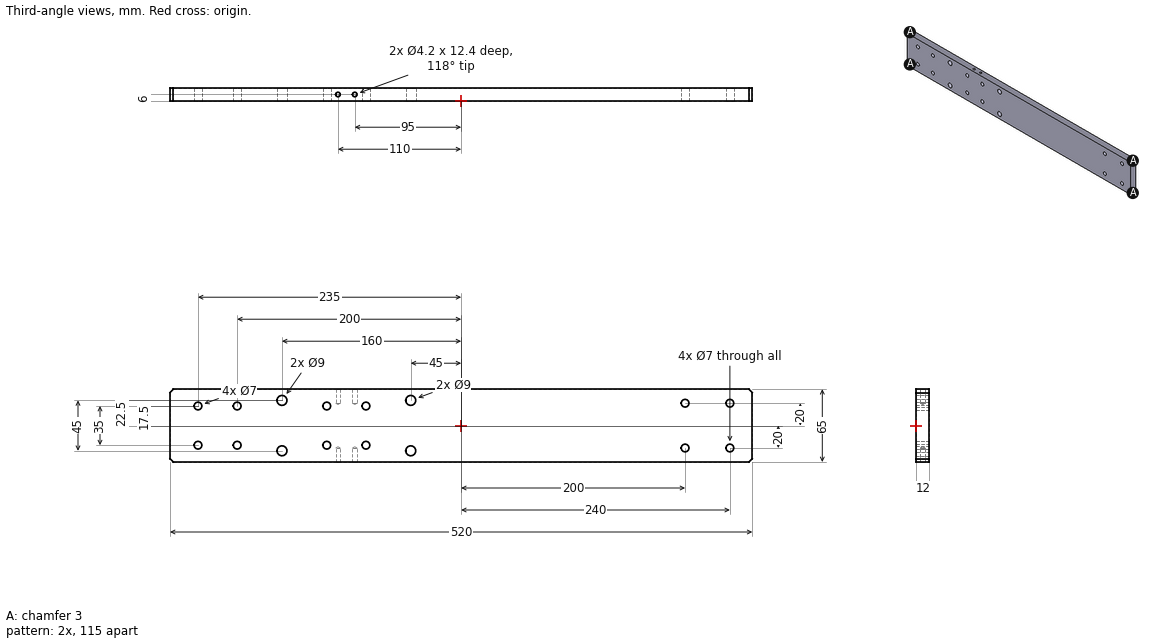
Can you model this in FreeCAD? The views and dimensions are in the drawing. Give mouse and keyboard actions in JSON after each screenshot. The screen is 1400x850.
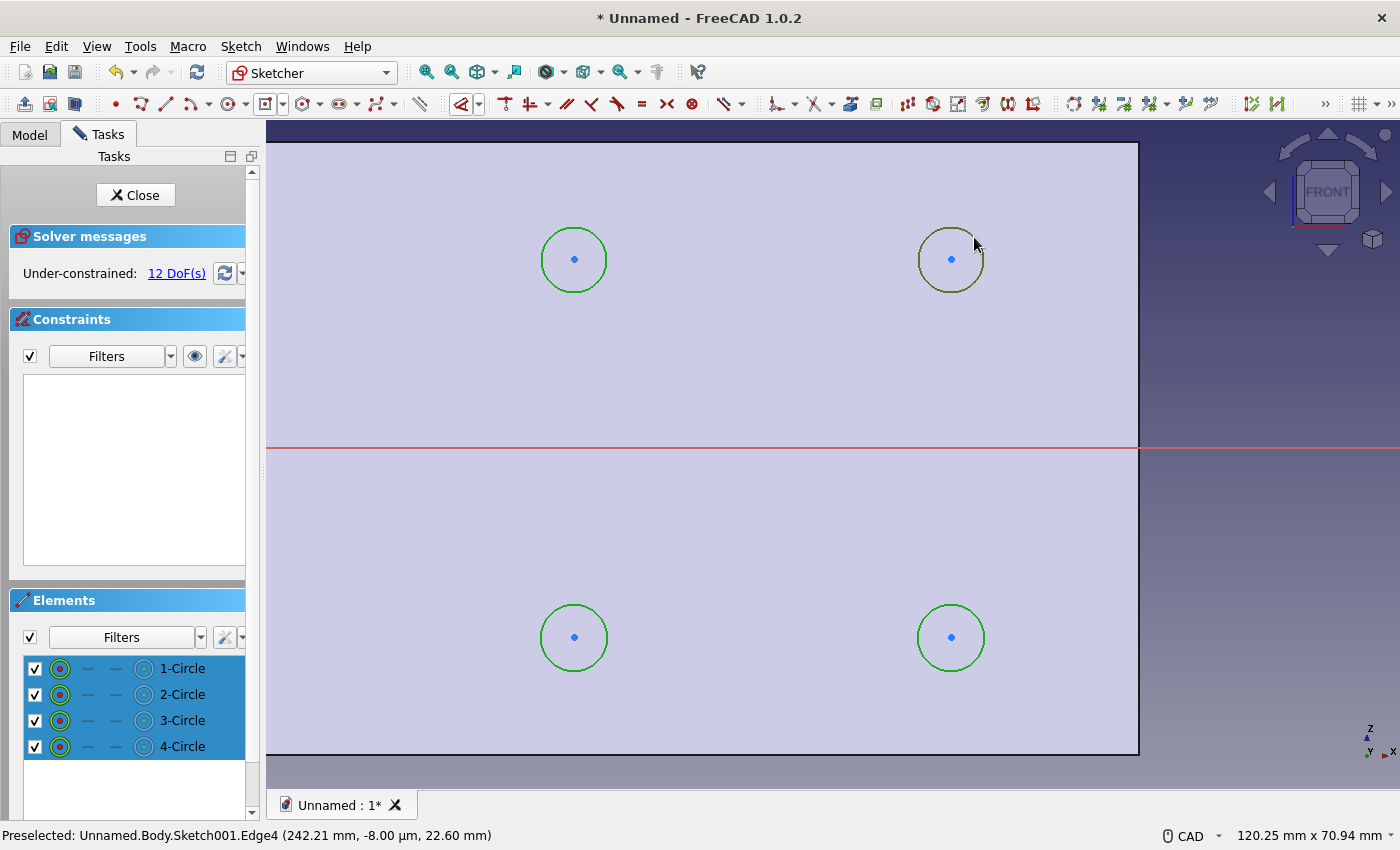
{"action": "left_click", "coordinate": [642, 104]}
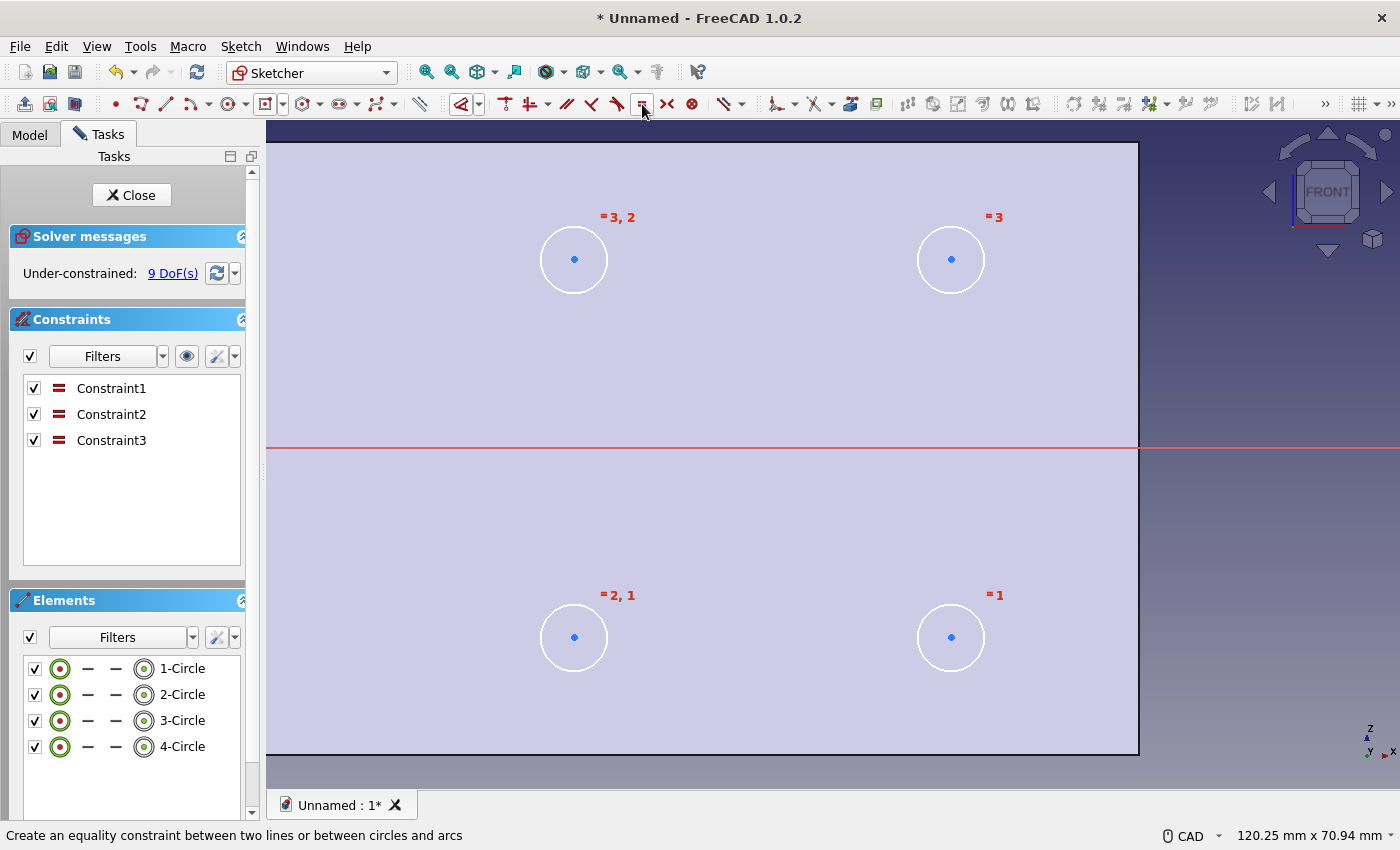
{"action": "left_click", "coordinate": [951, 638]}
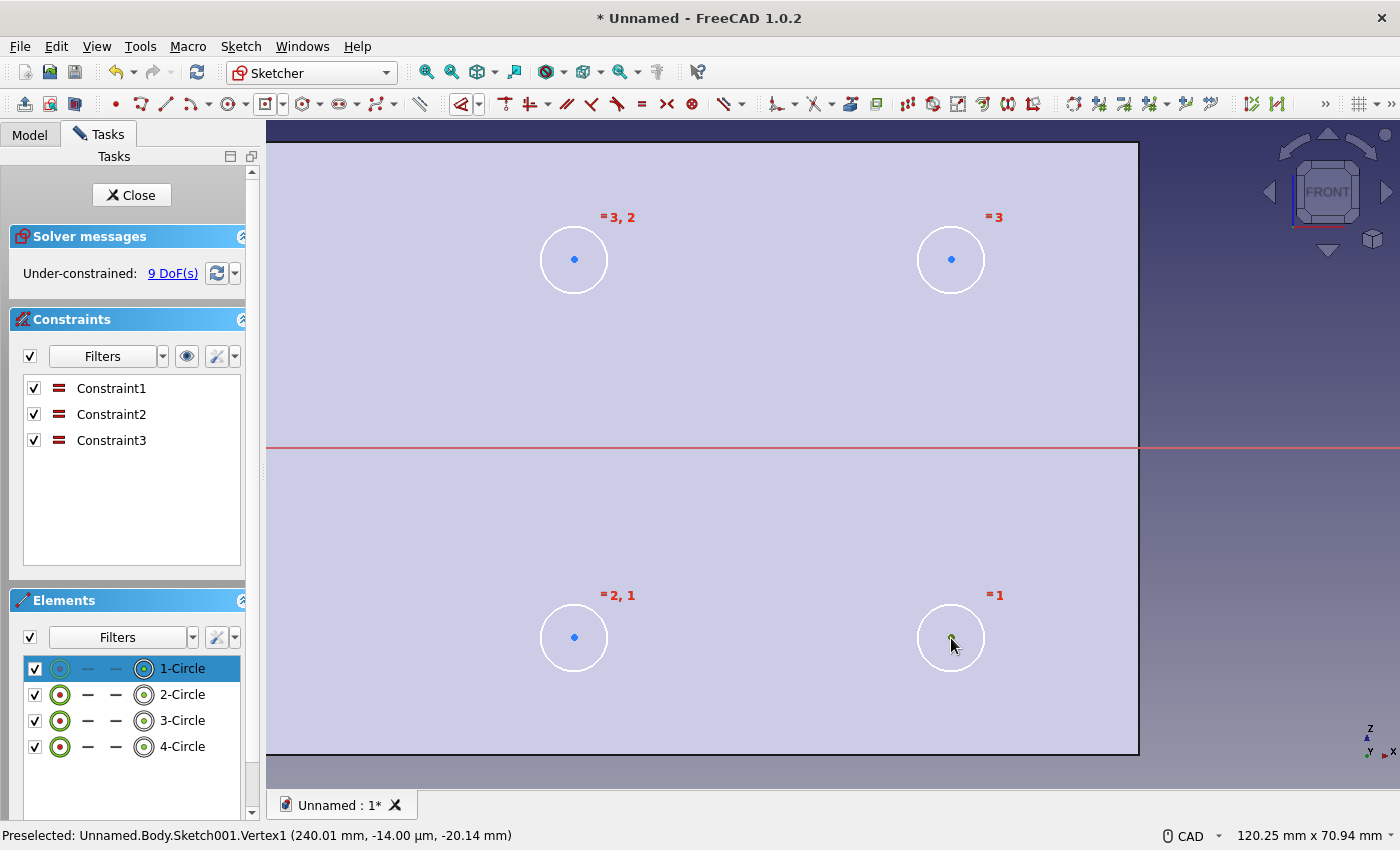
{"action": "left_click", "coordinate": [574, 638]}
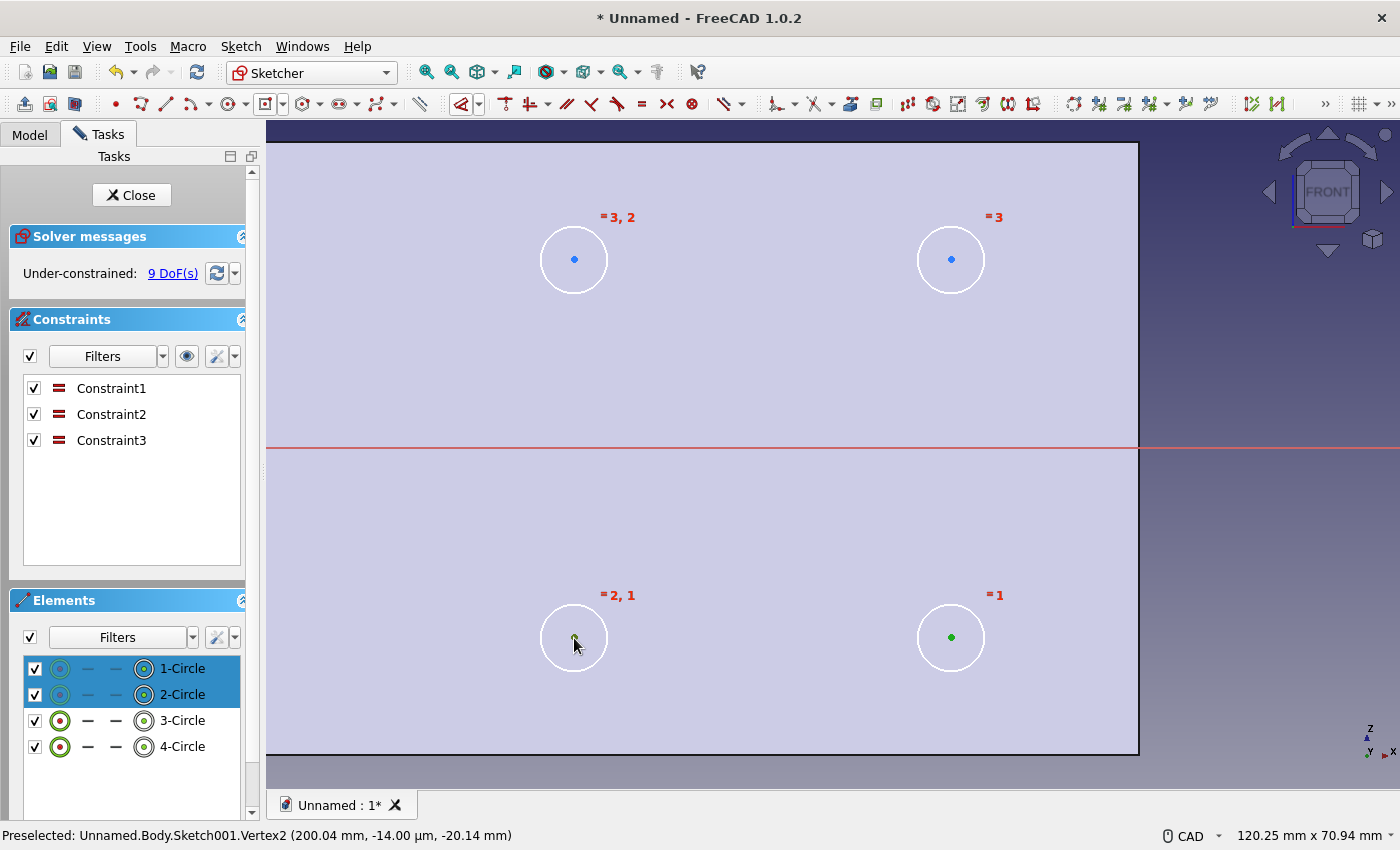
{"action": "key", "text": "h"}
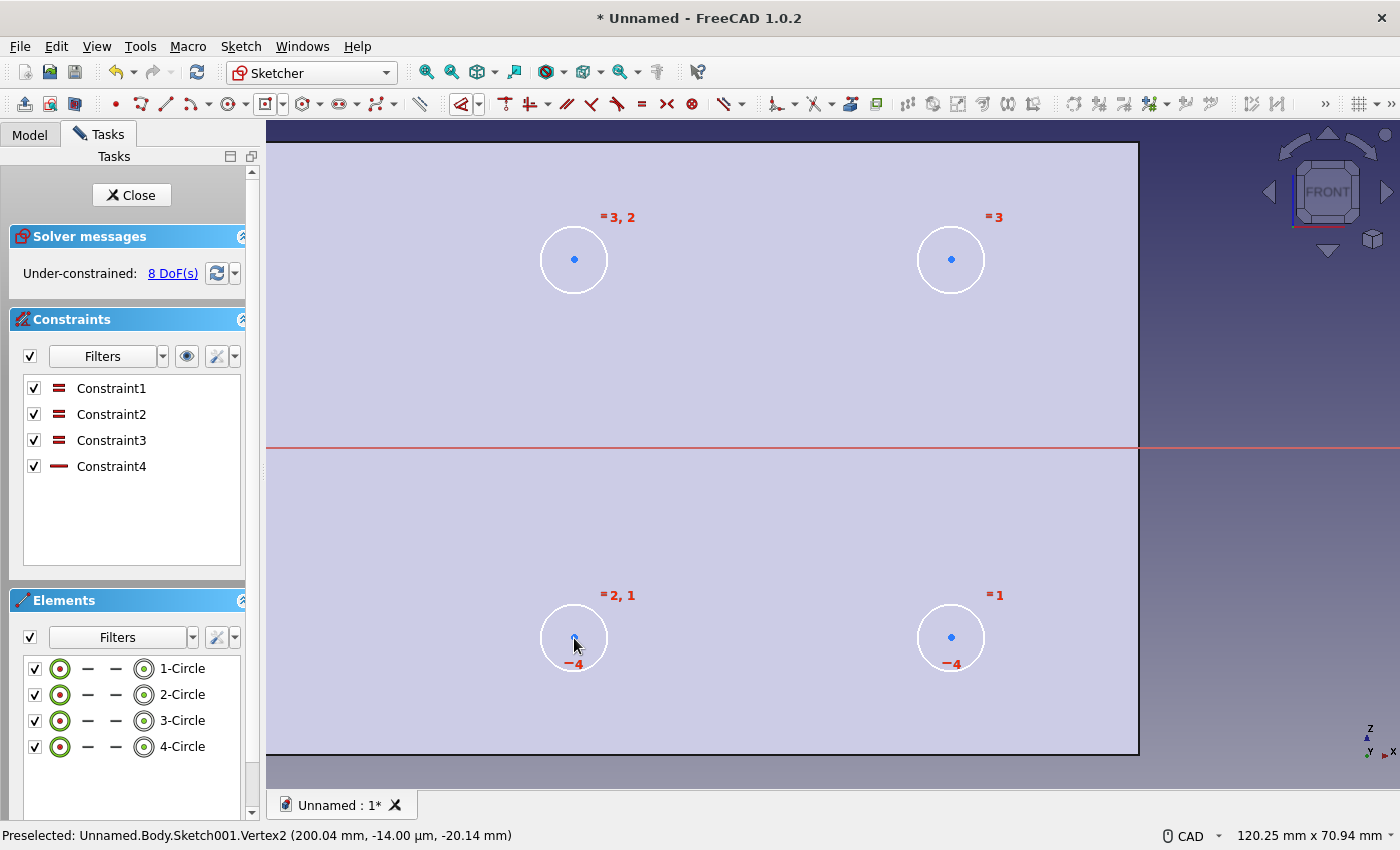
{"action": "left_click", "coordinate": [574, 638]}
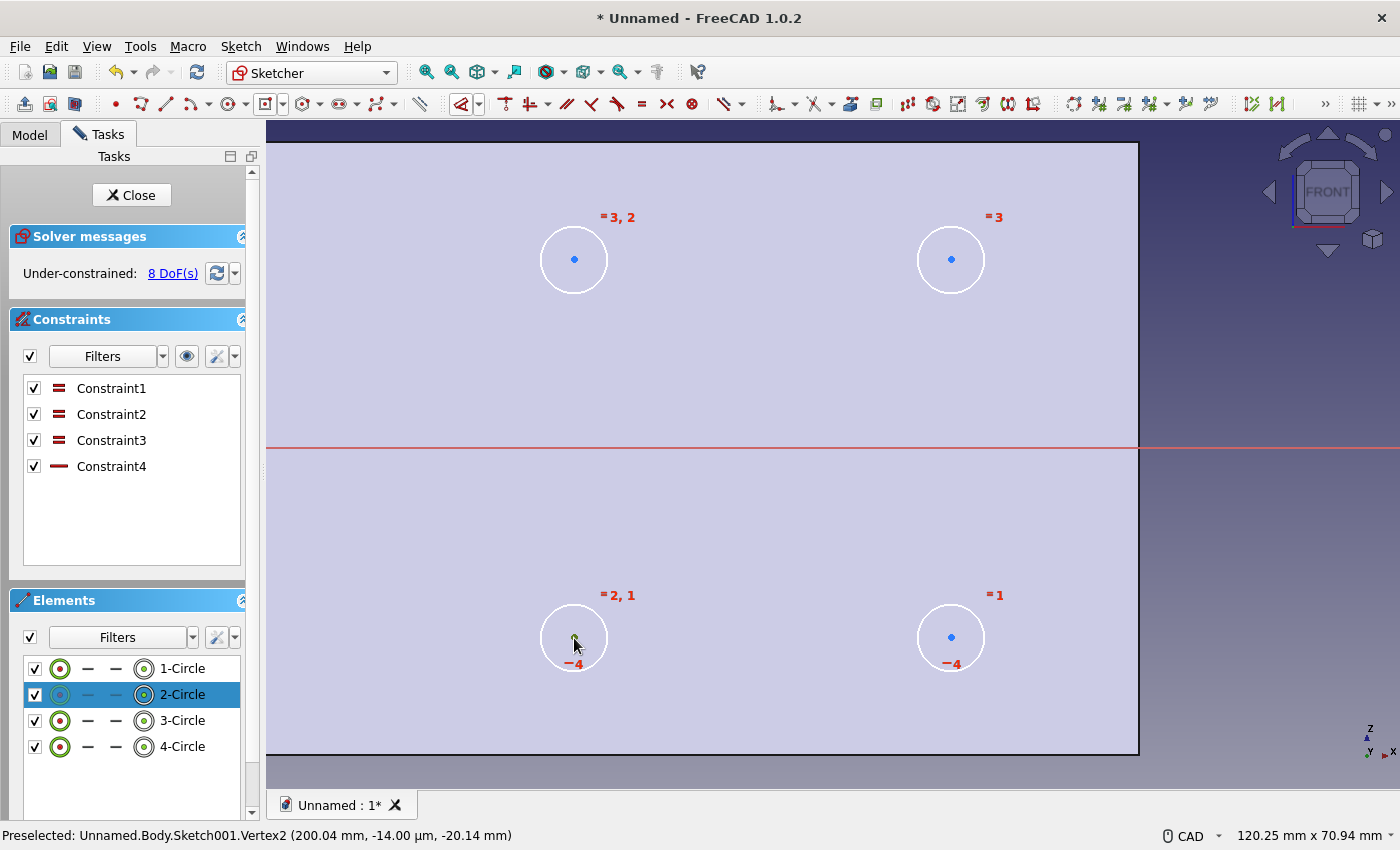
{"action": "left_click", "coordinate": [574, 260]}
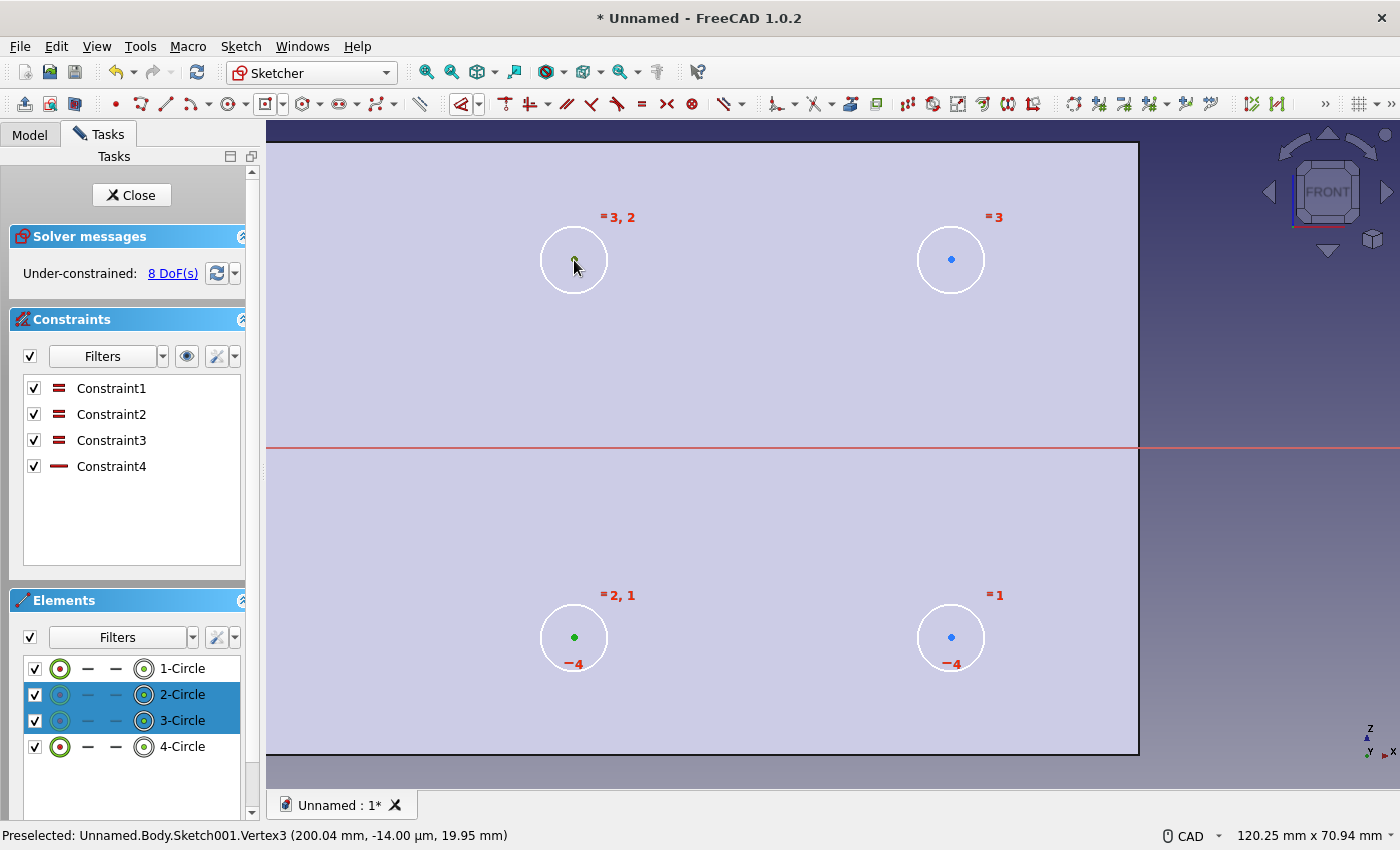
{"action": "key", "text": "v"}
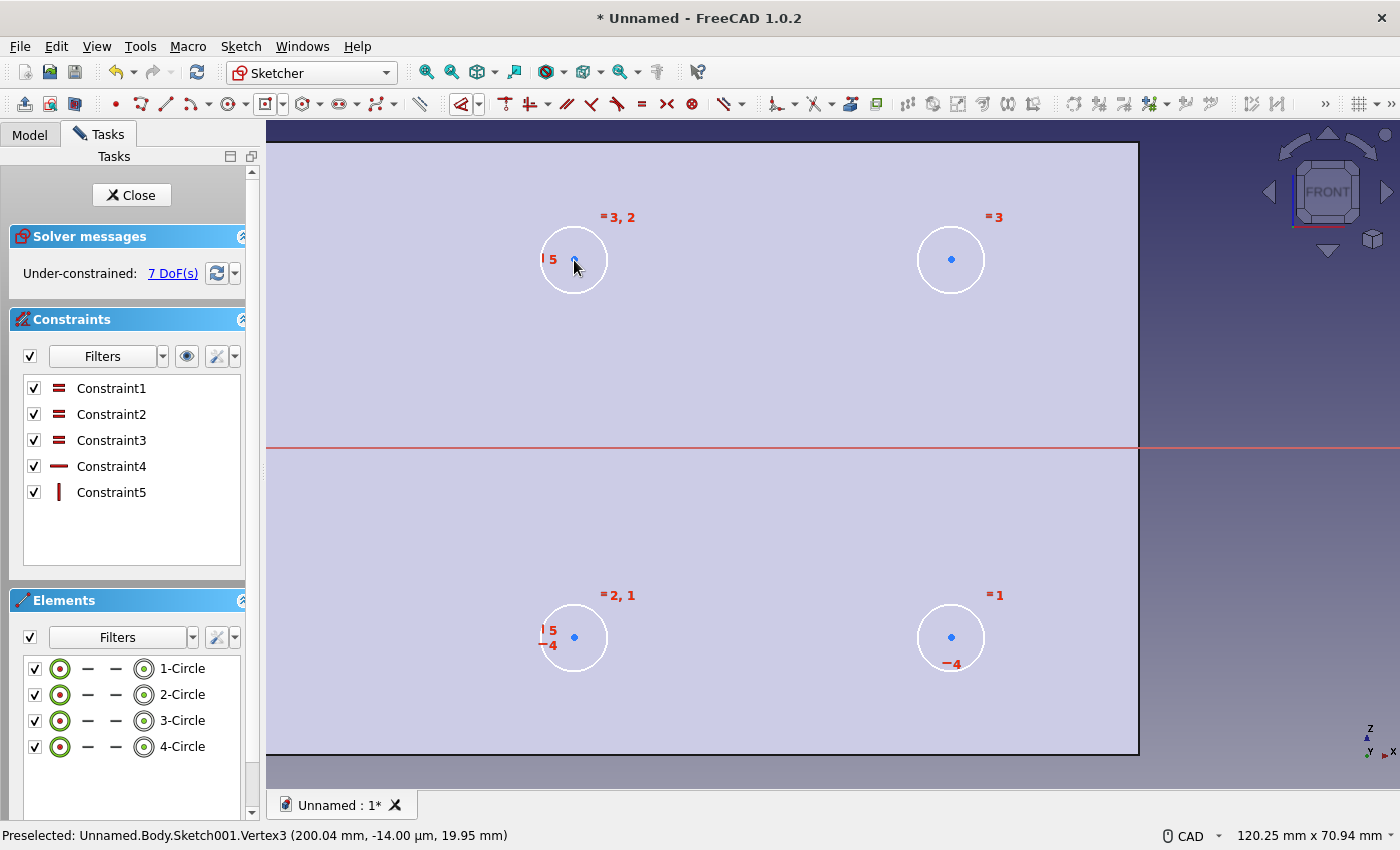
{"action": "left_click", "coordinate": [951, 638]}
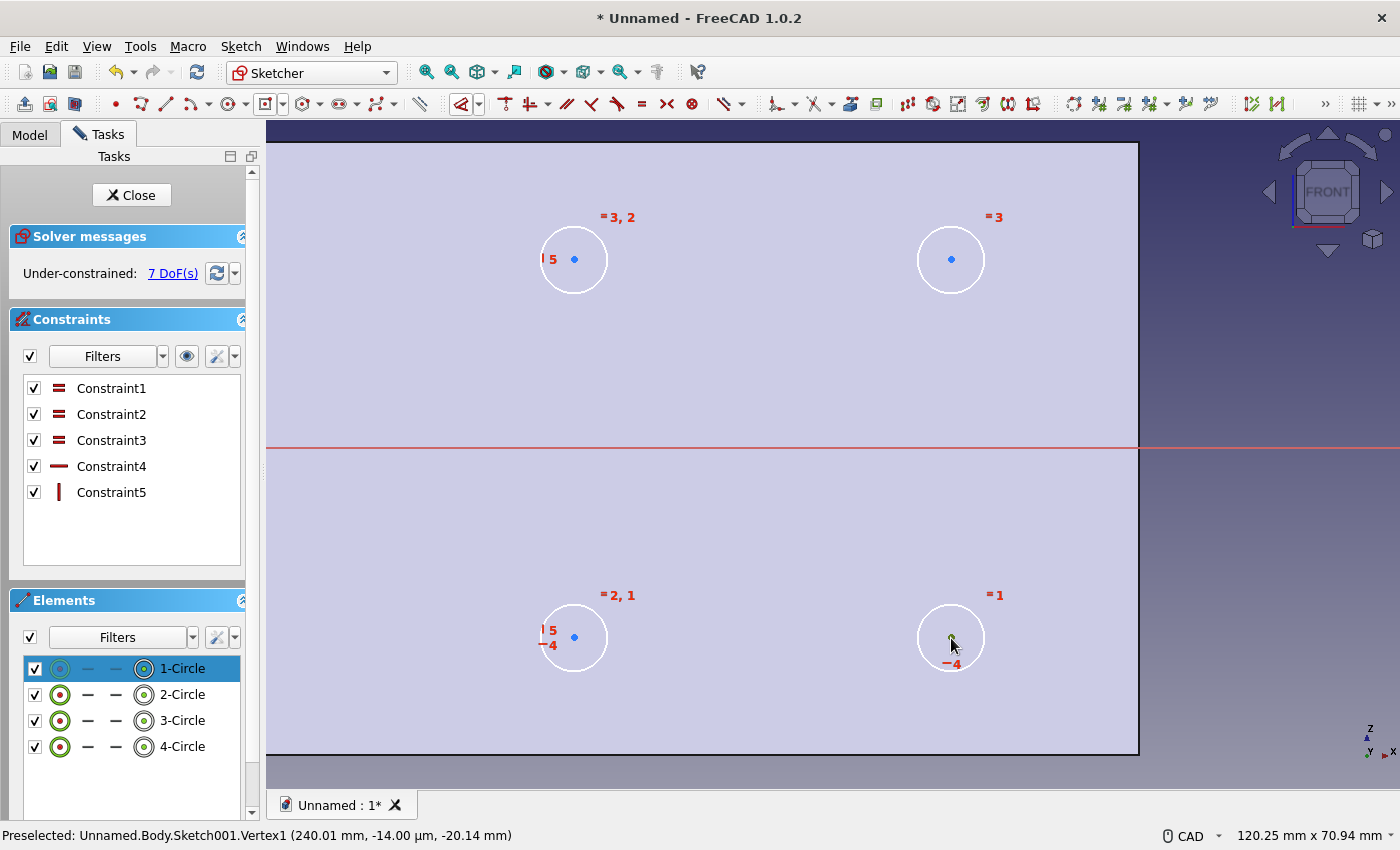
{"action": "left_click", "coordinate": [951, 260]}